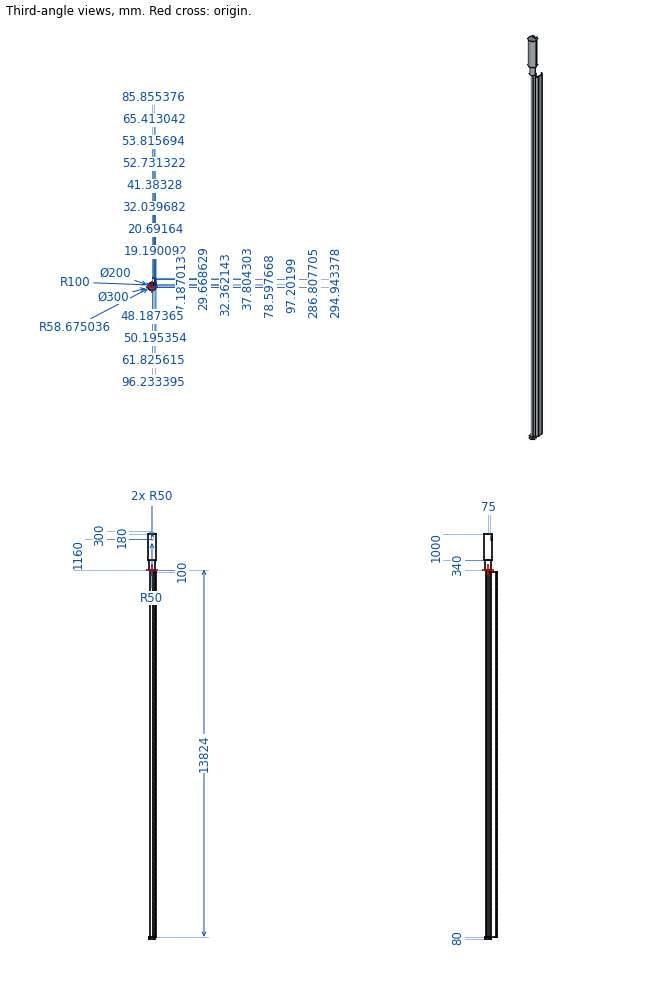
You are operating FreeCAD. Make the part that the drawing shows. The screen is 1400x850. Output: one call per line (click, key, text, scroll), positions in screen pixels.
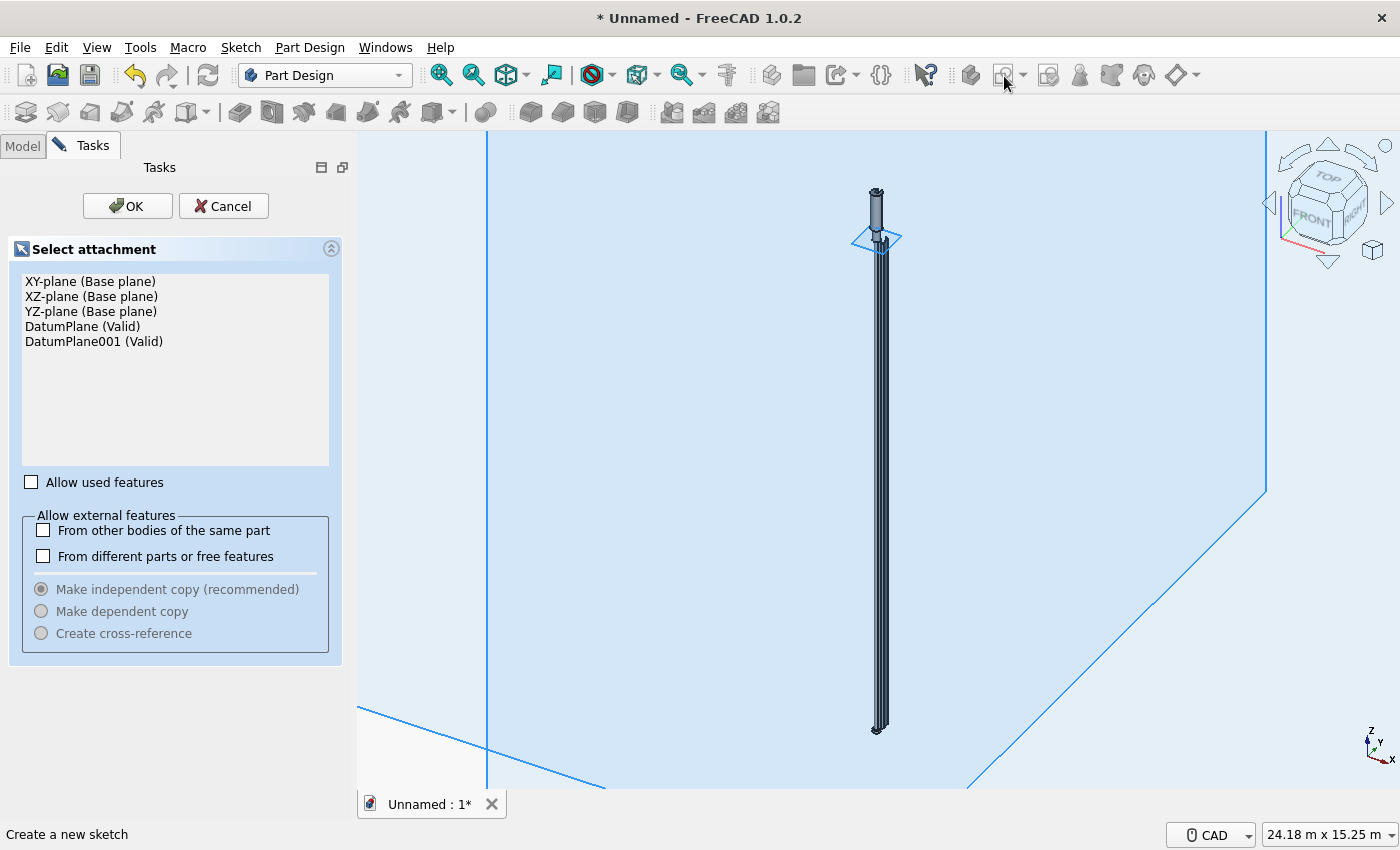
click(82, 296)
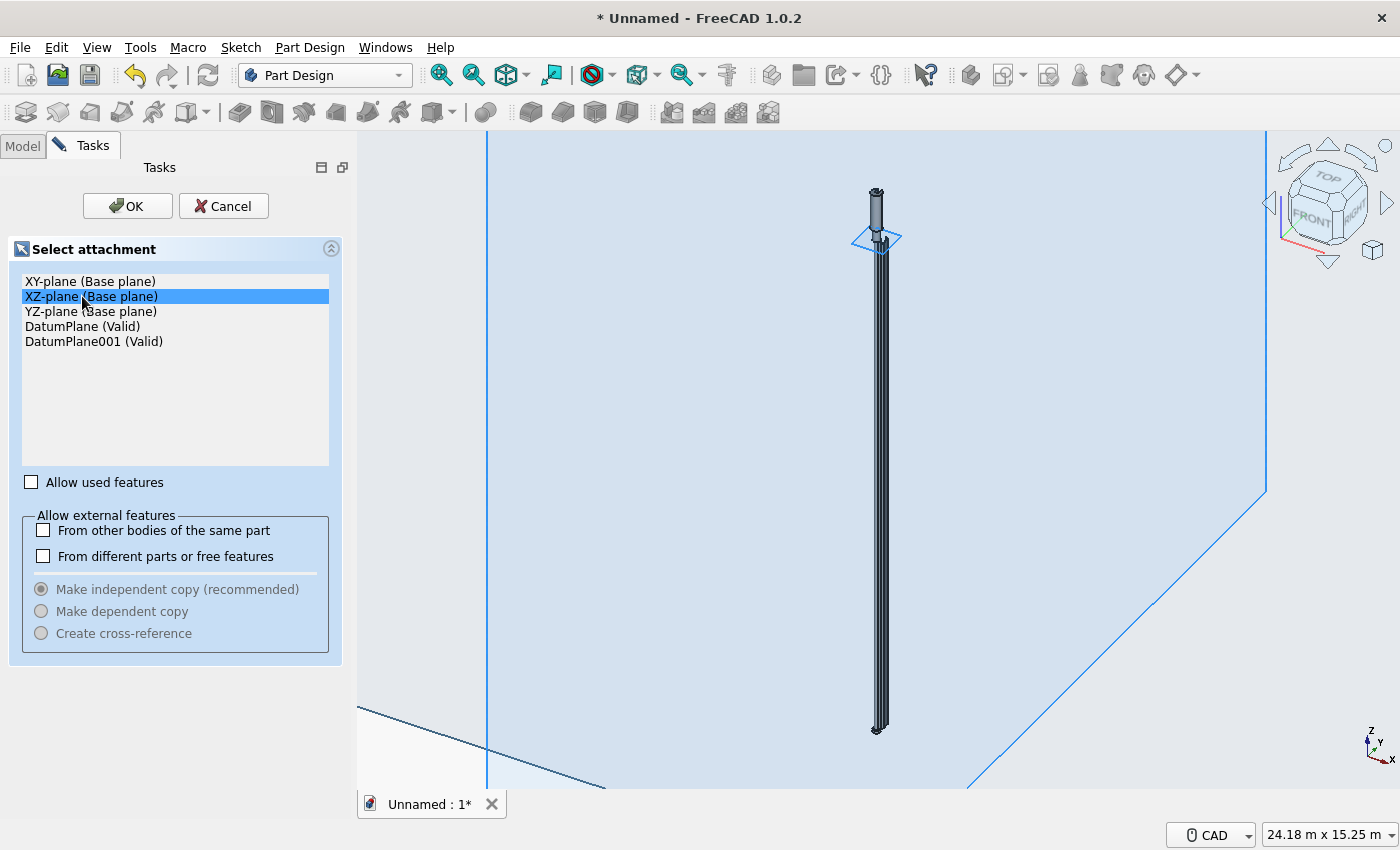
click(128, 206)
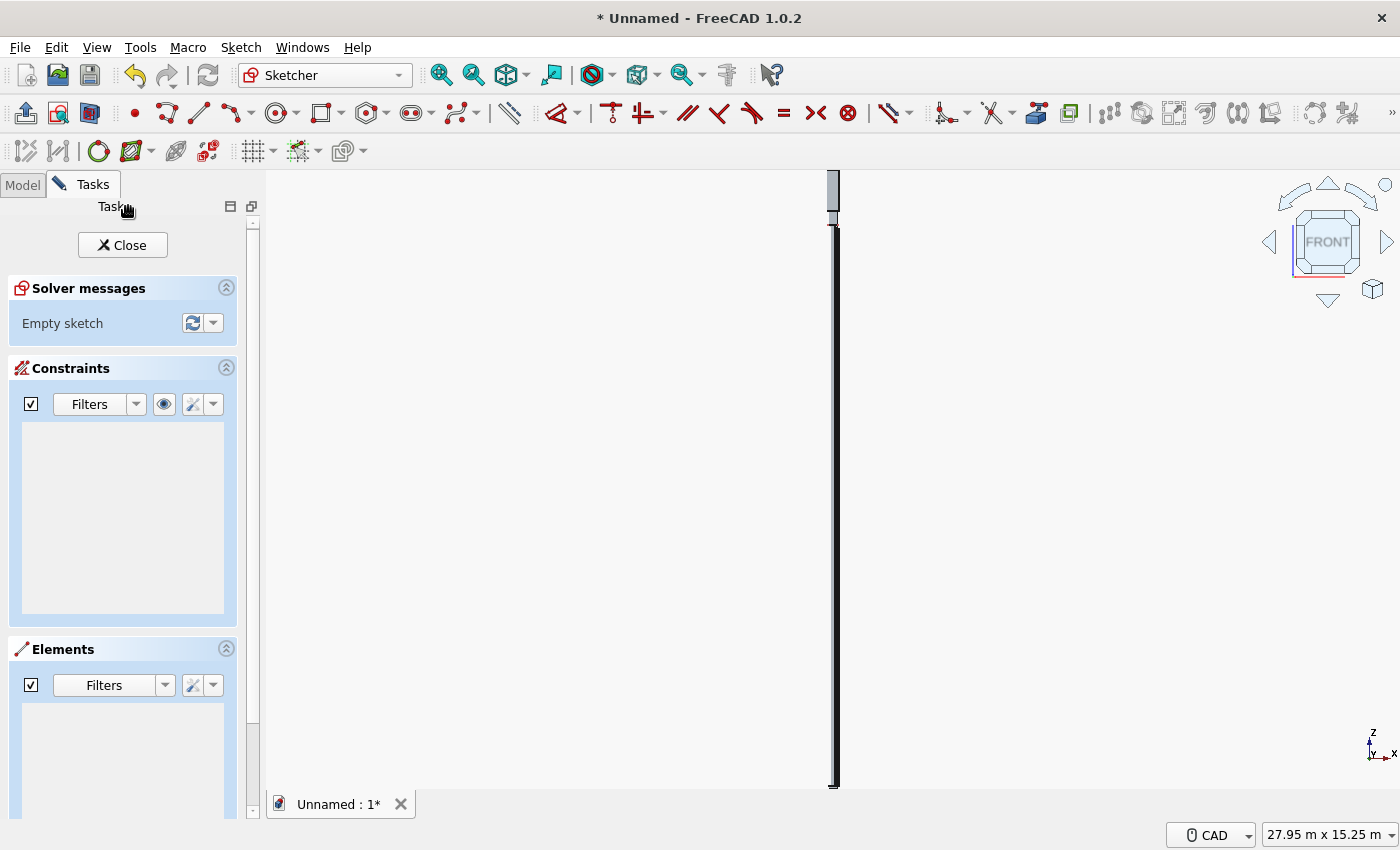
key(q)
key(s)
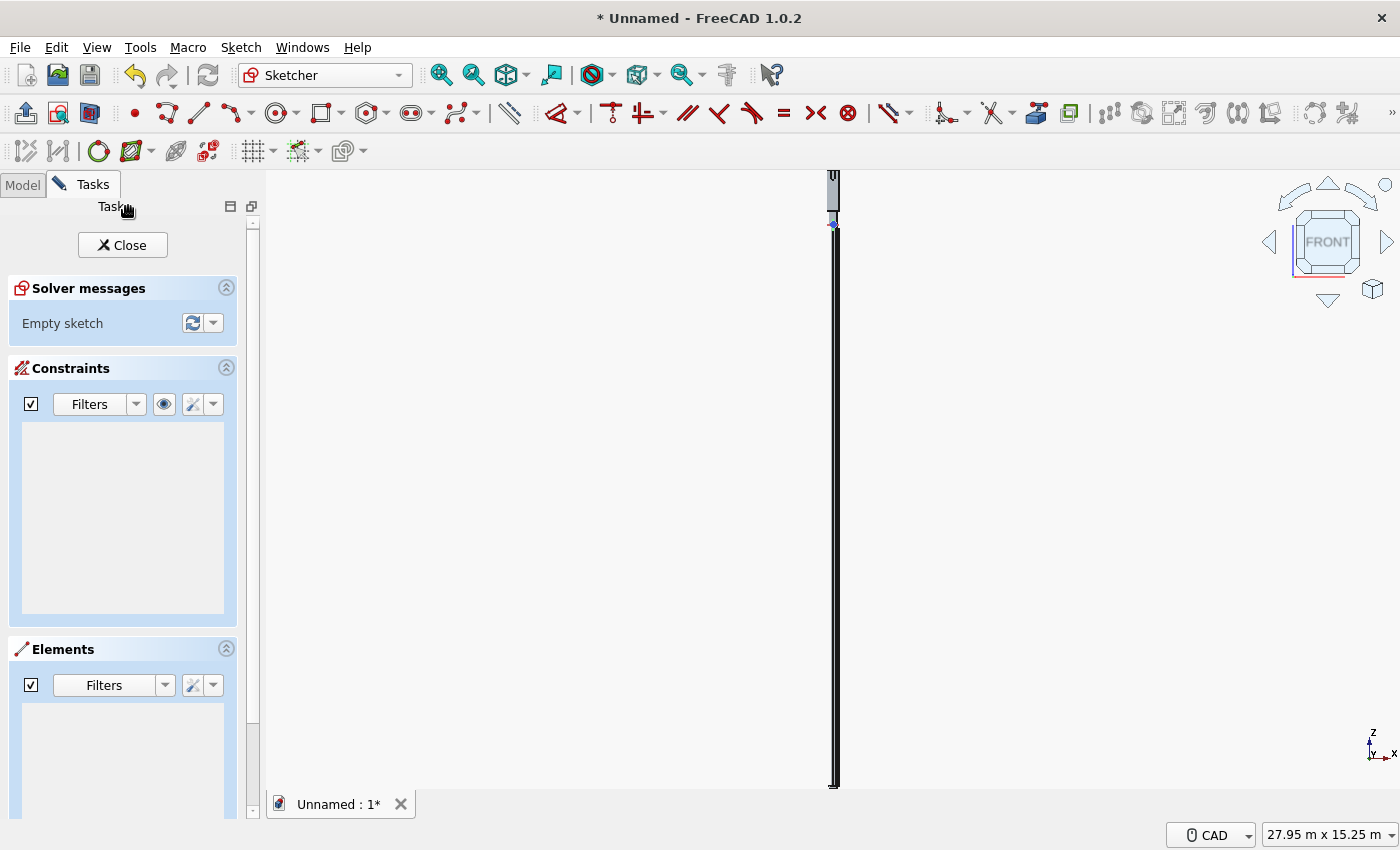
scroll(764, 480, down, 5)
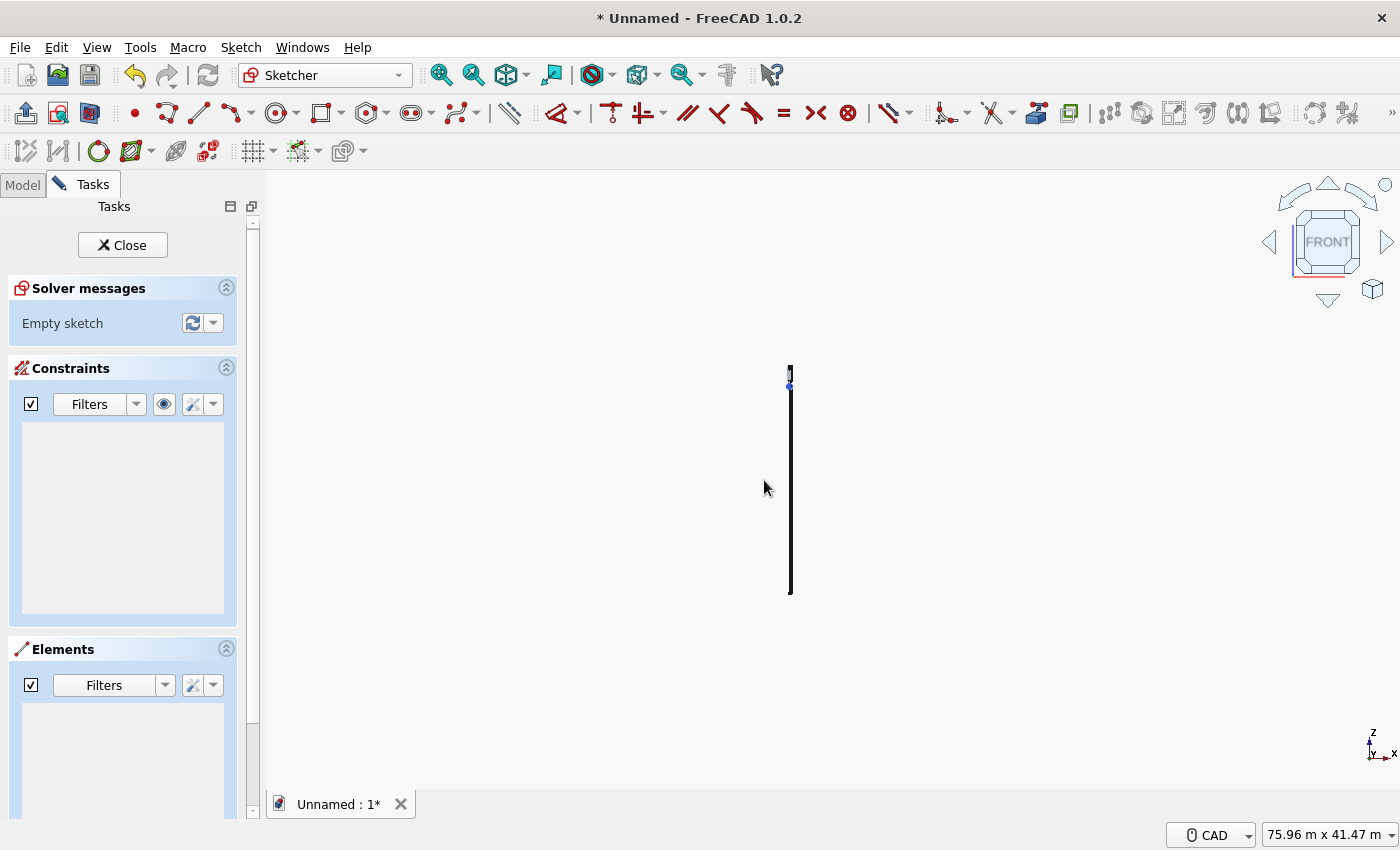
scroll(791, 362, up, 15)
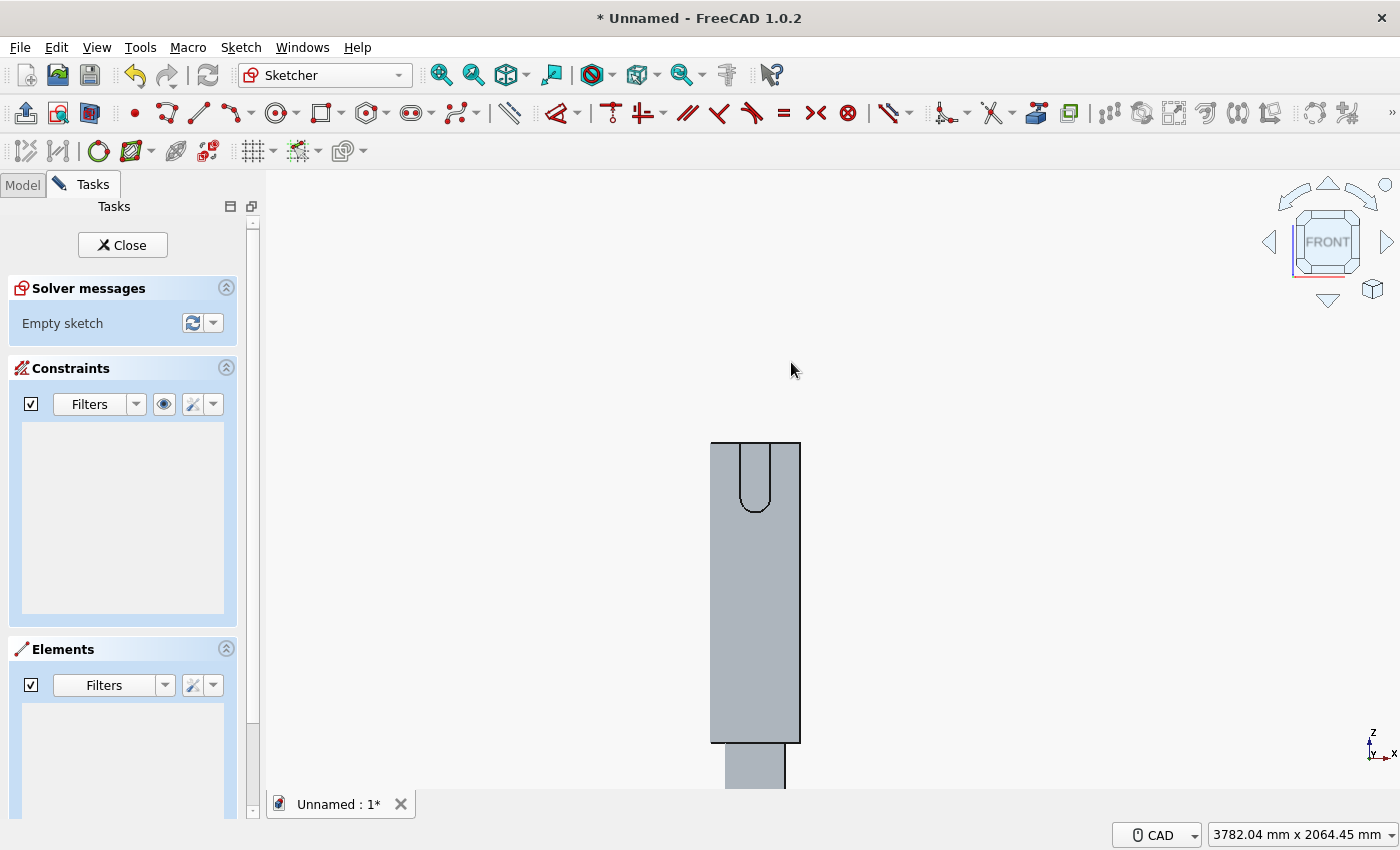
scroll(753, 478, up, 9)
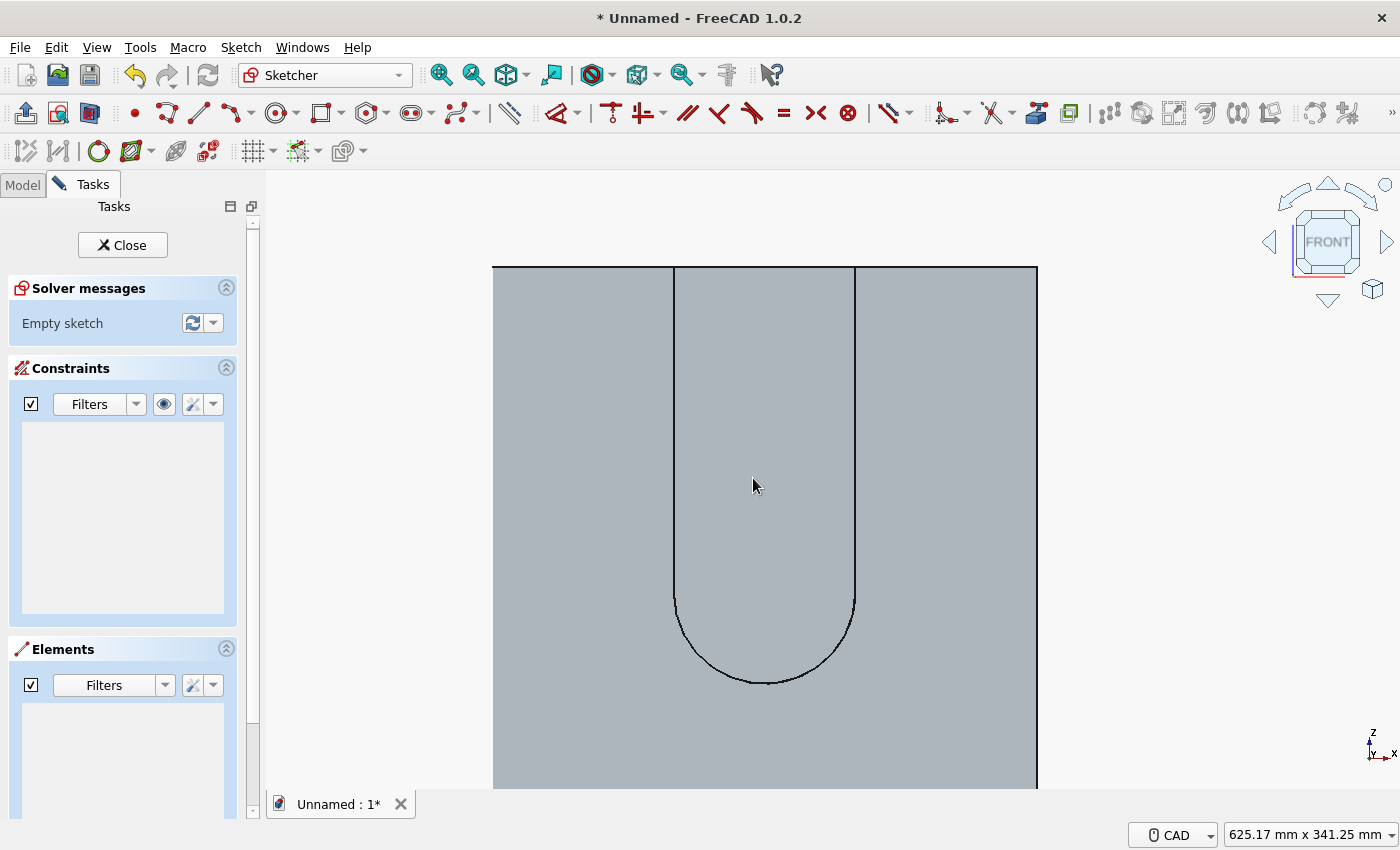
key(g)
key(m)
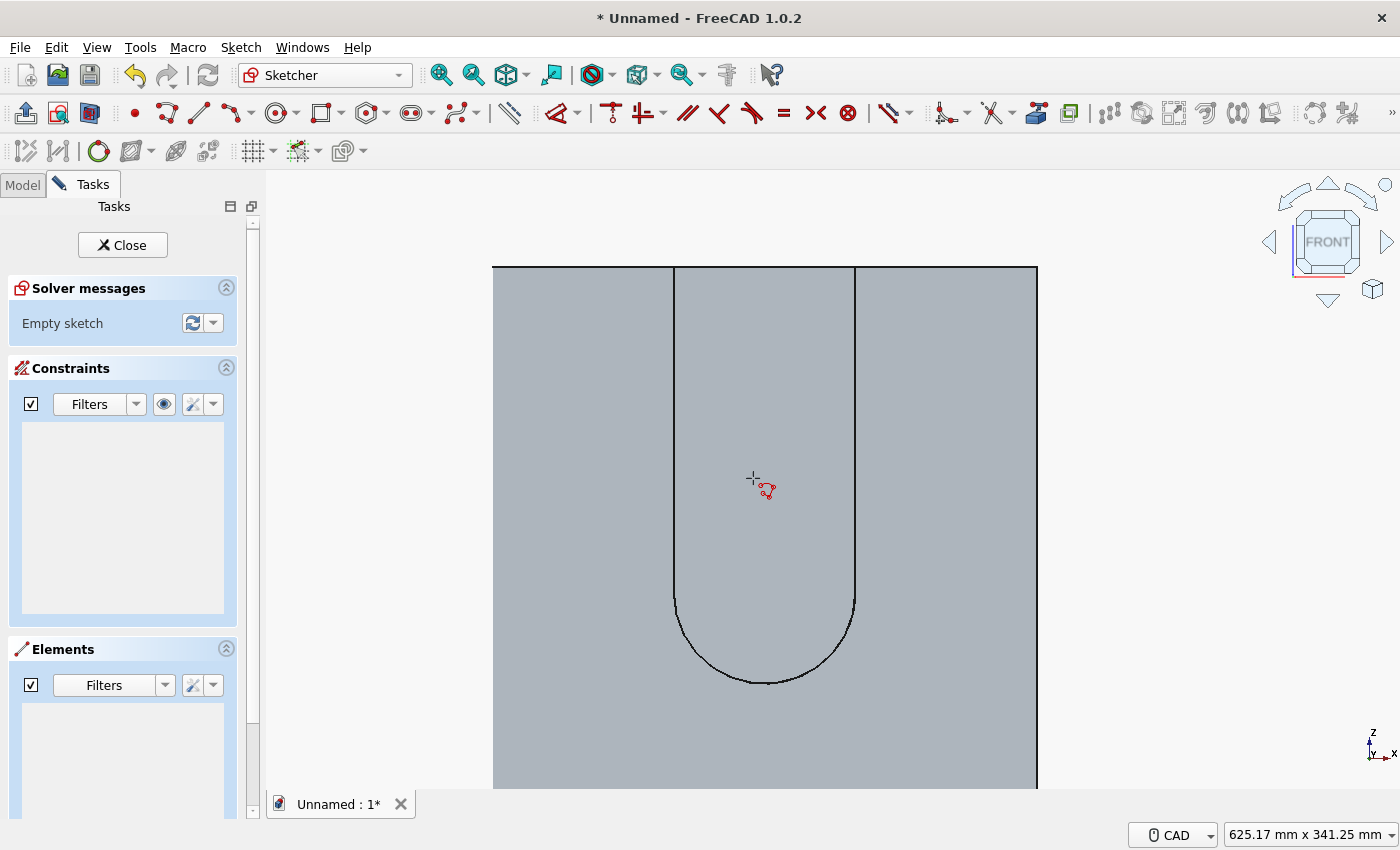
click(674, 593)
click(674, 267)
click(855, 267)
click(855, 593)
right_click(855, 593)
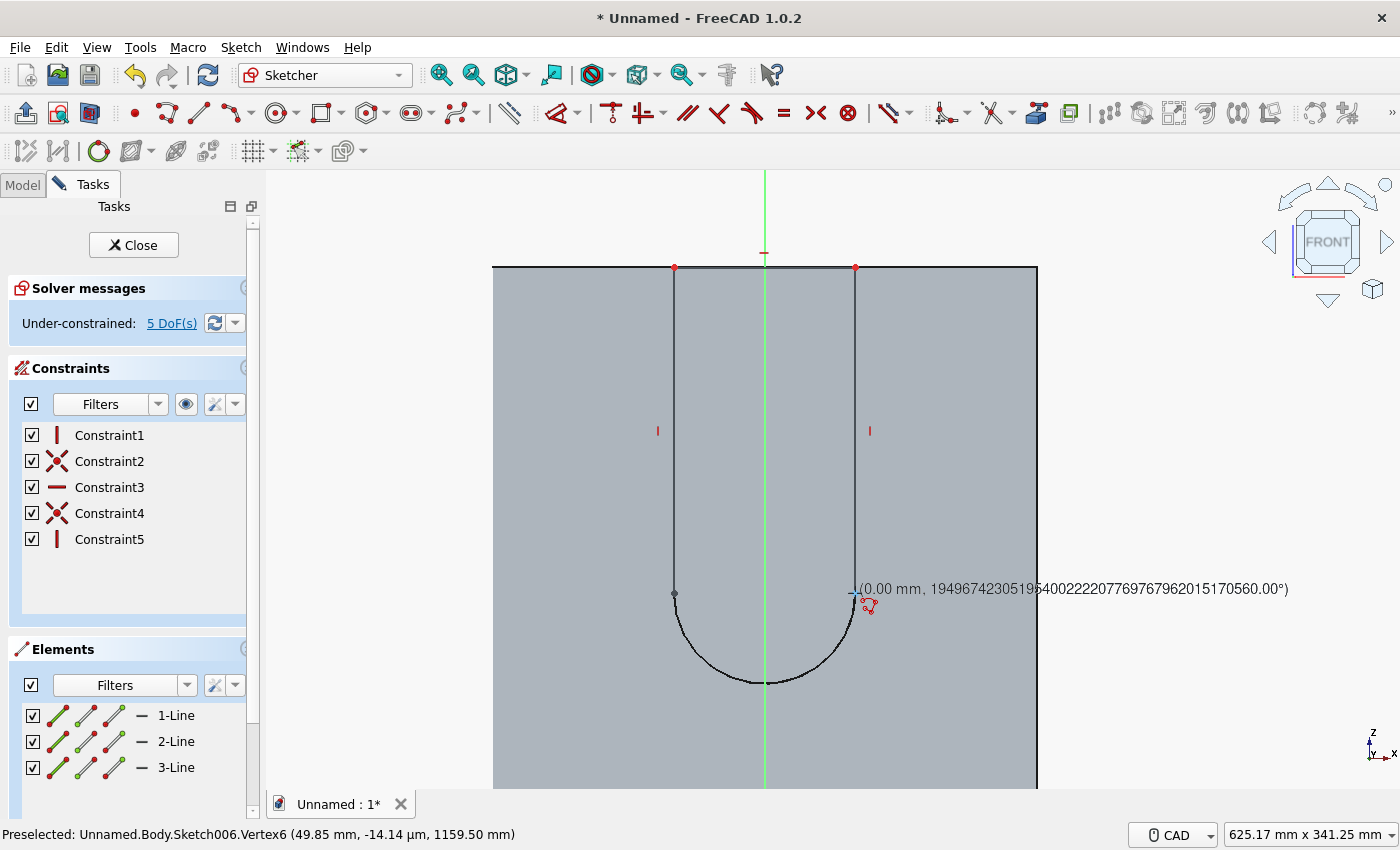
key(g)
key(3)
key(a)